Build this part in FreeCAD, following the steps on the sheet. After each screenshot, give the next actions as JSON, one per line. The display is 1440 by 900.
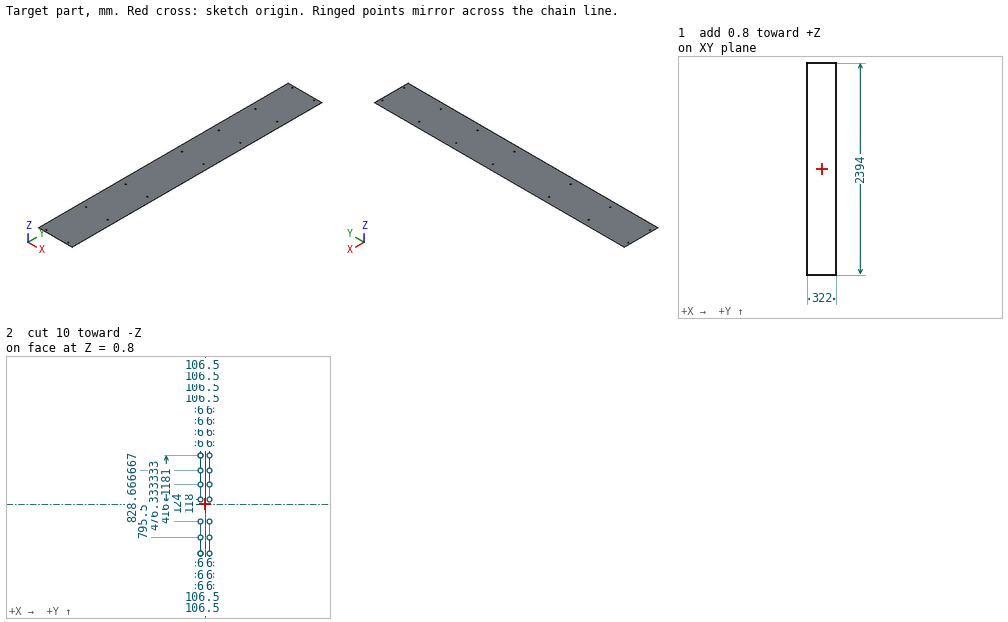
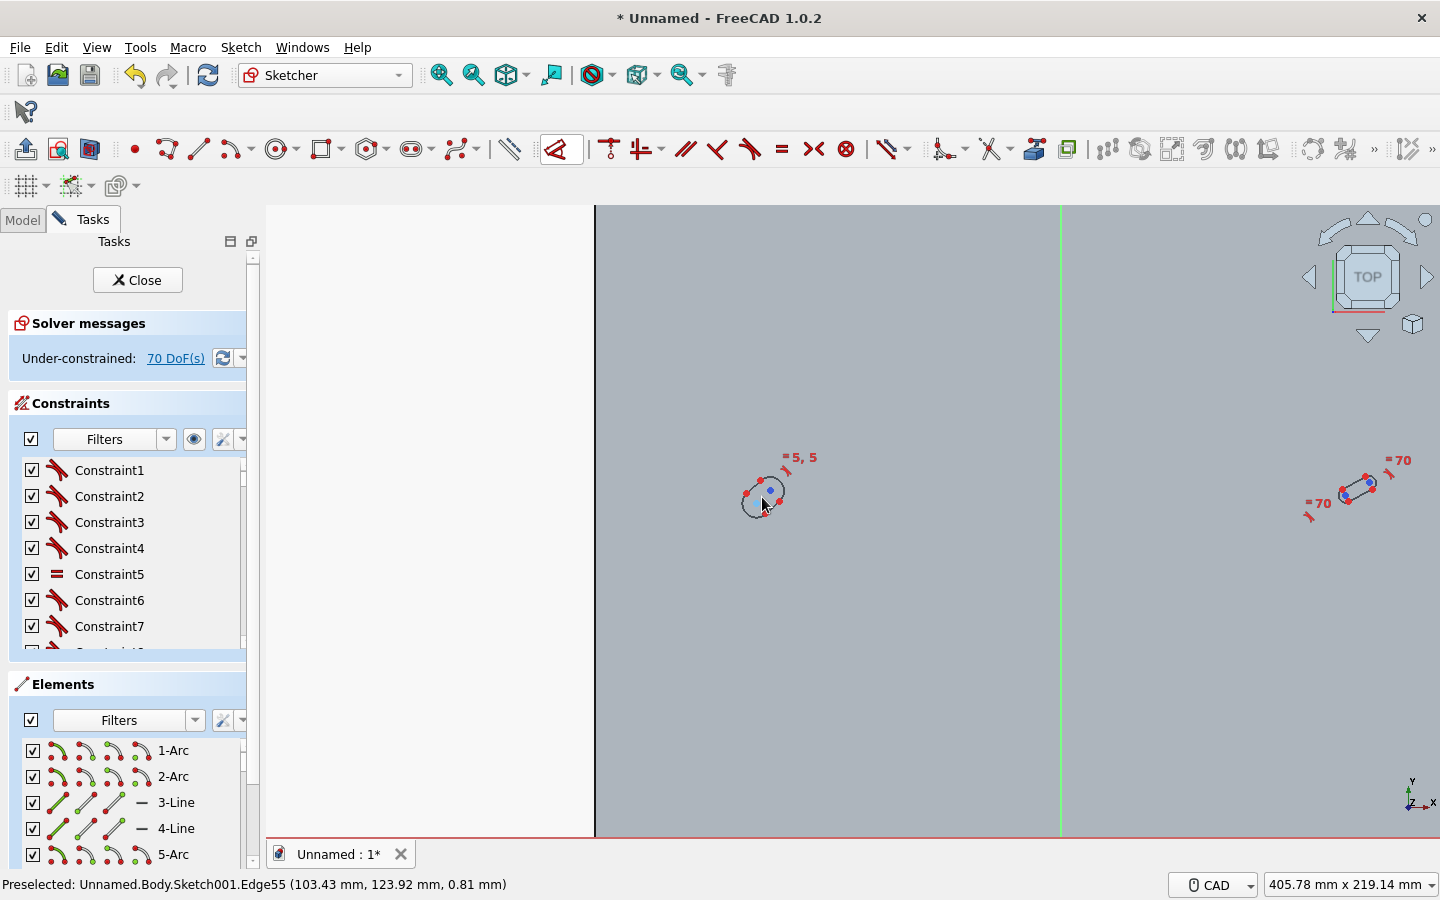
{"action": "left_click", "coordinate": [757, 485]}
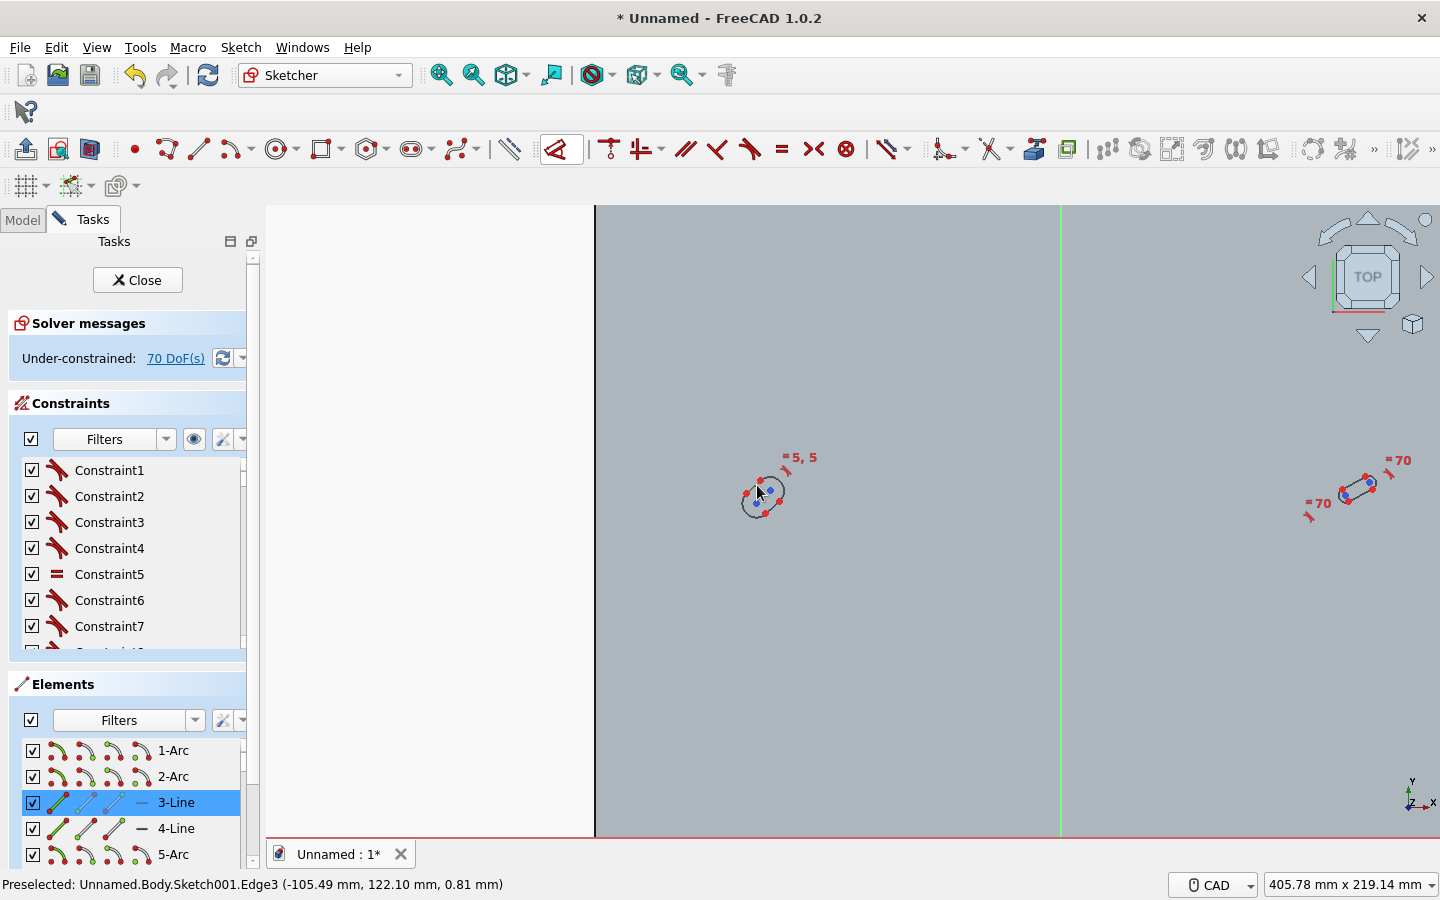
{"action": "key", "text": "h"}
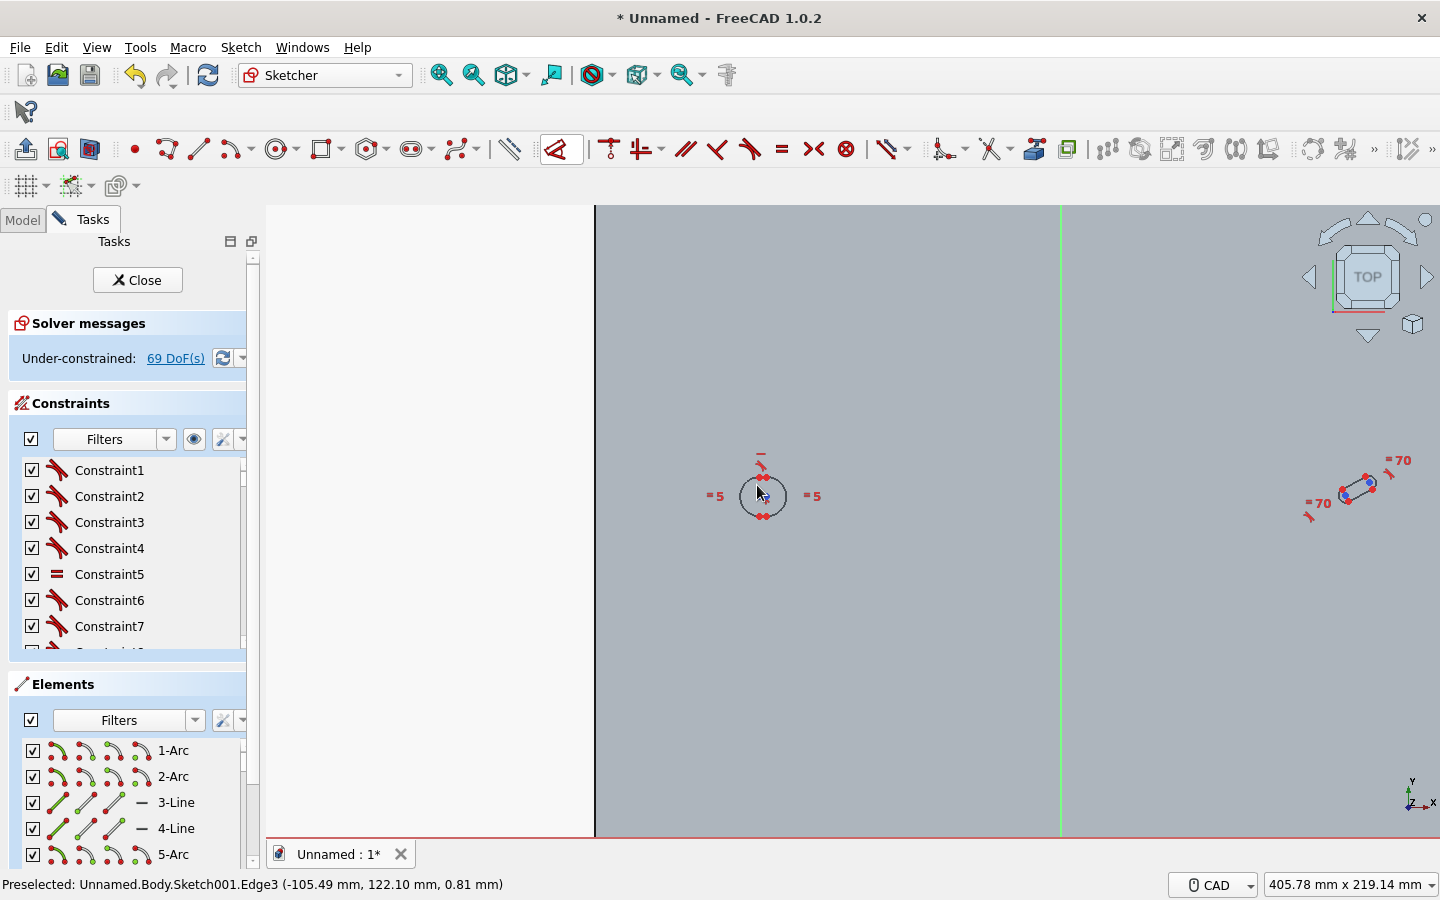
{"action": "scroll", "coordinate": [767, 502], "scroll_direction": "down", "scroll_amount": 14}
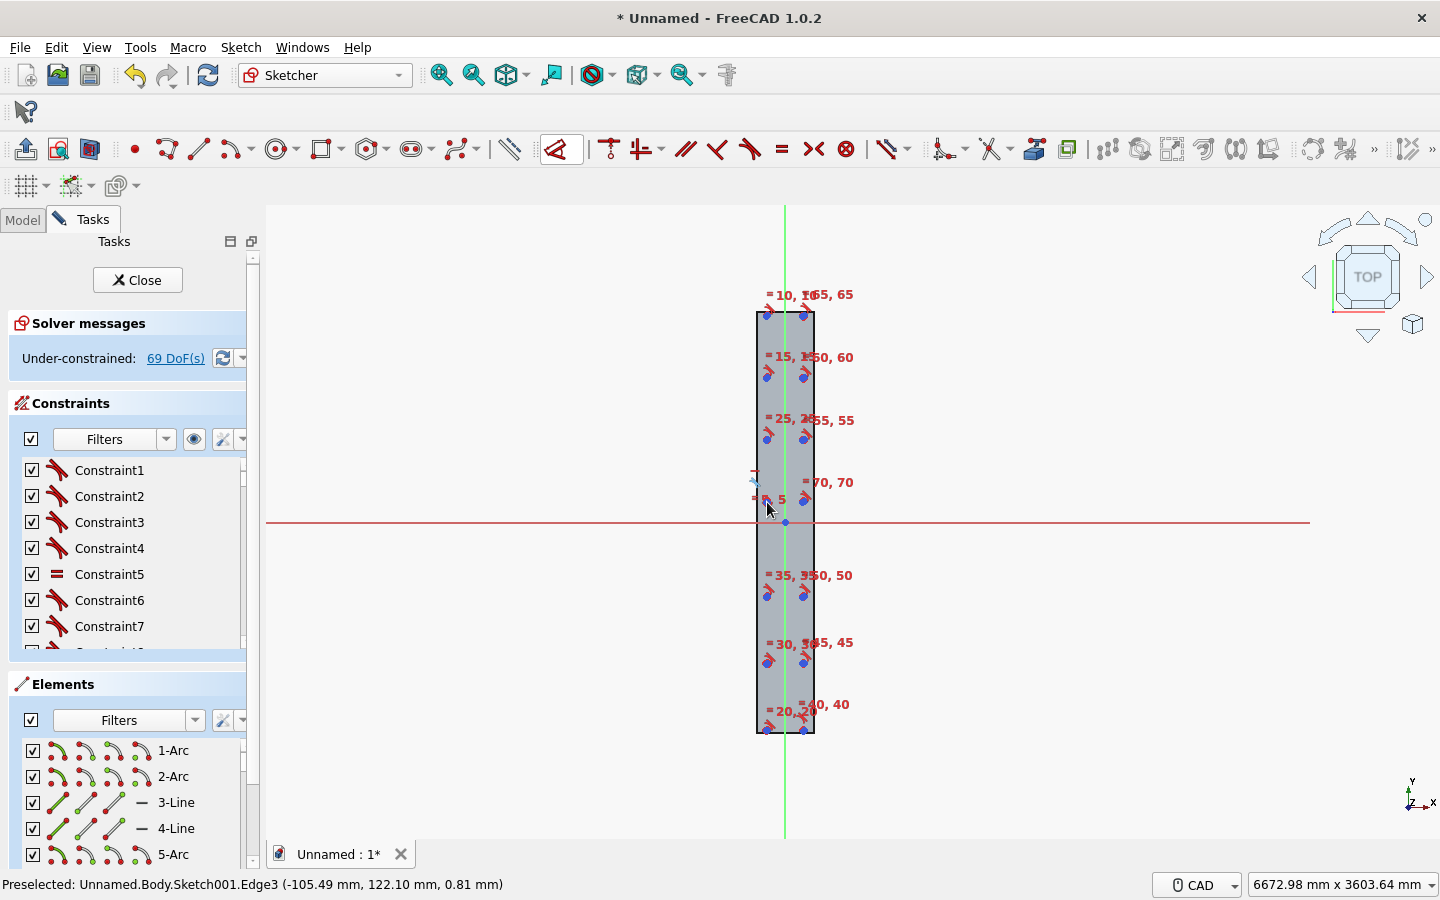
{"action": "scroll", "coordinate": [767, 315], "scroll_direction": "up", "scroll_amount": 14}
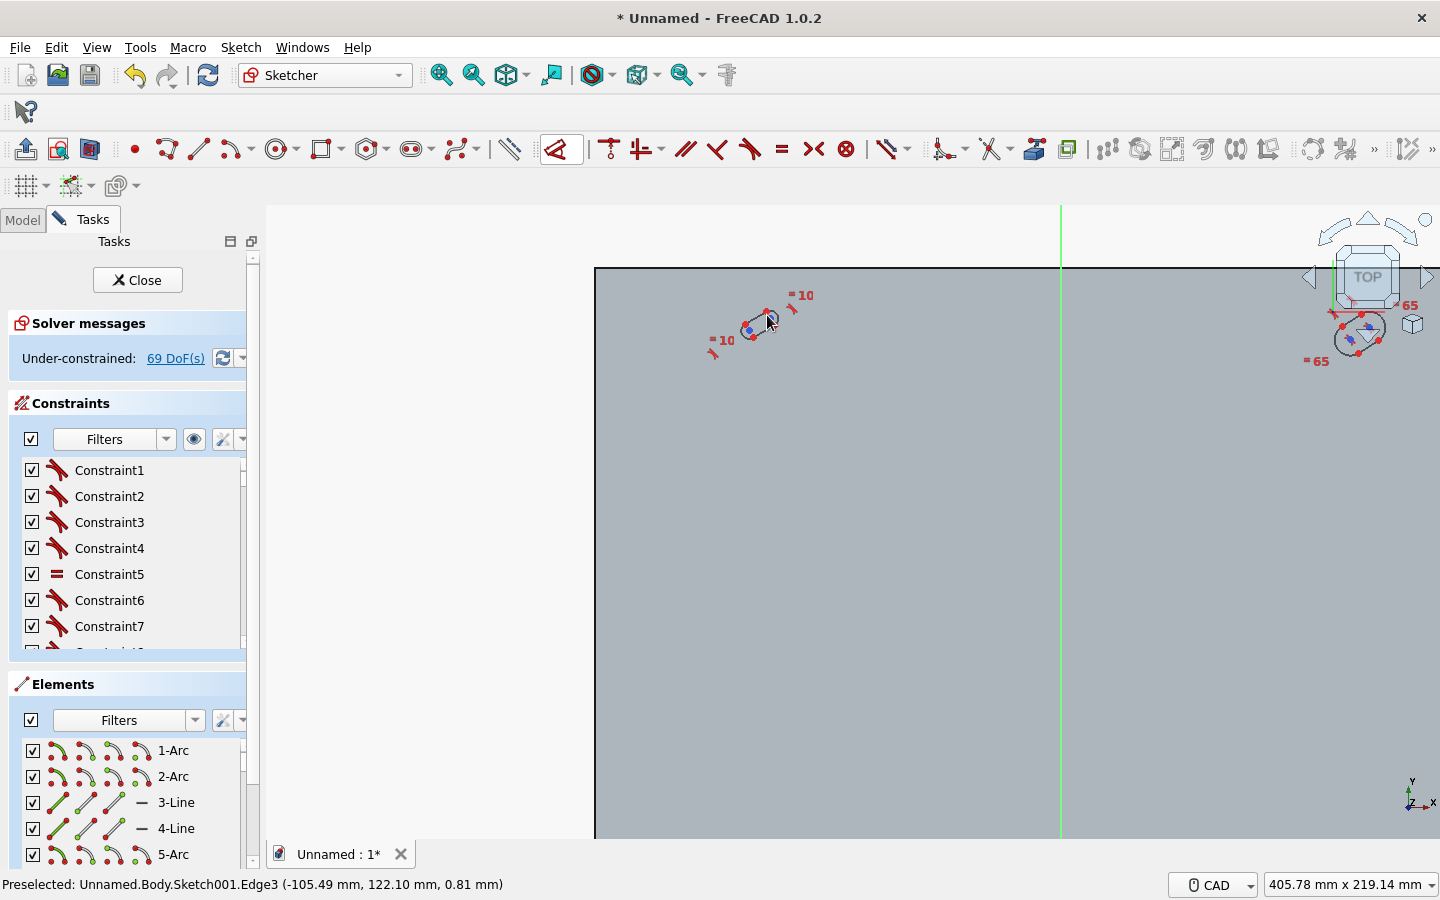
{"action": "left_click", "coordinate": [754, 319]}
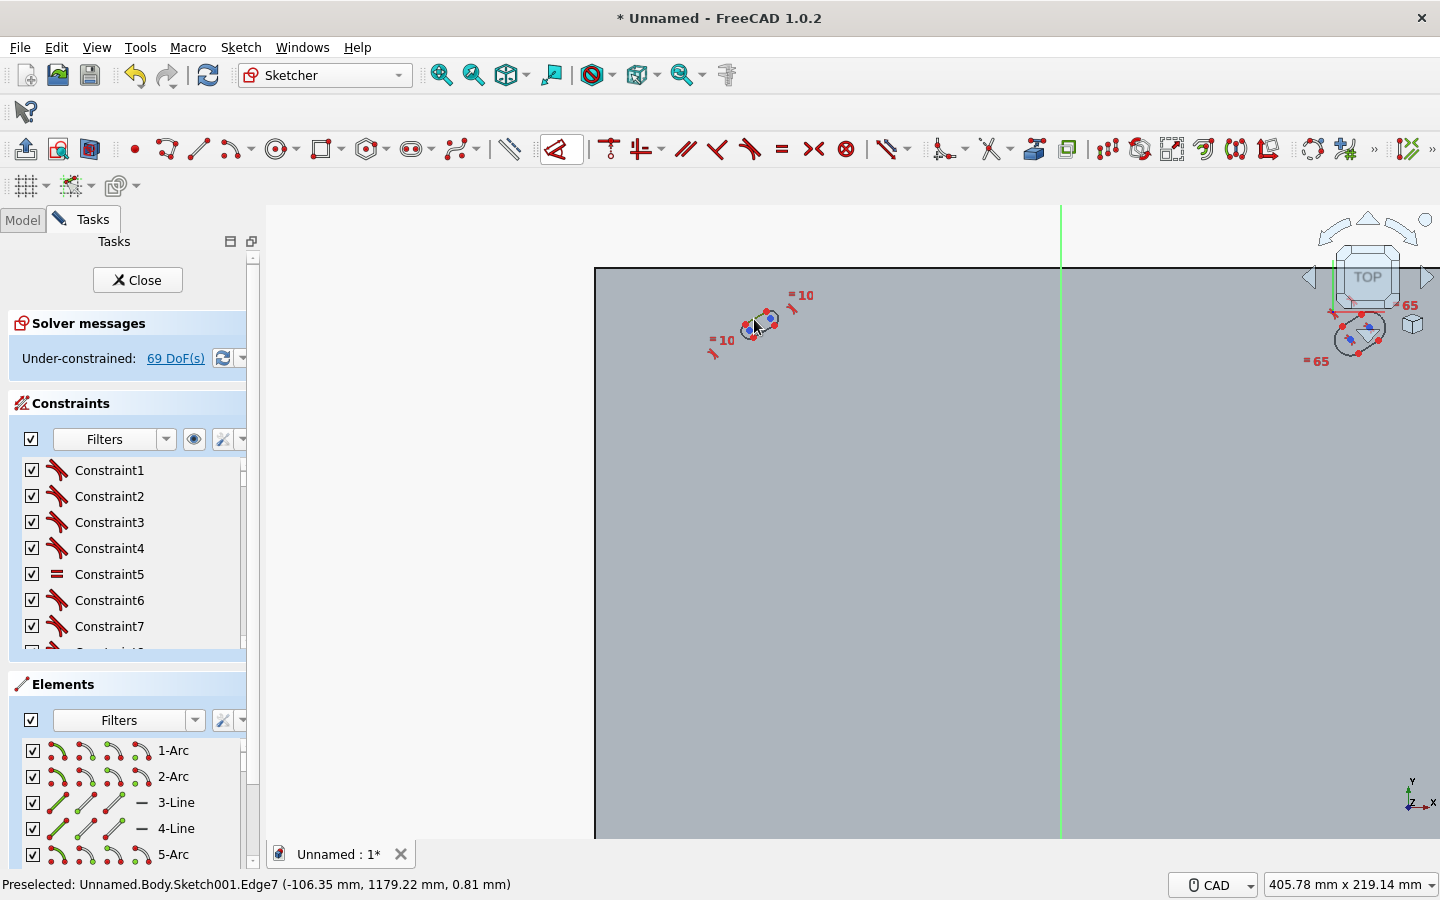
{"action": "key", "text": "h"}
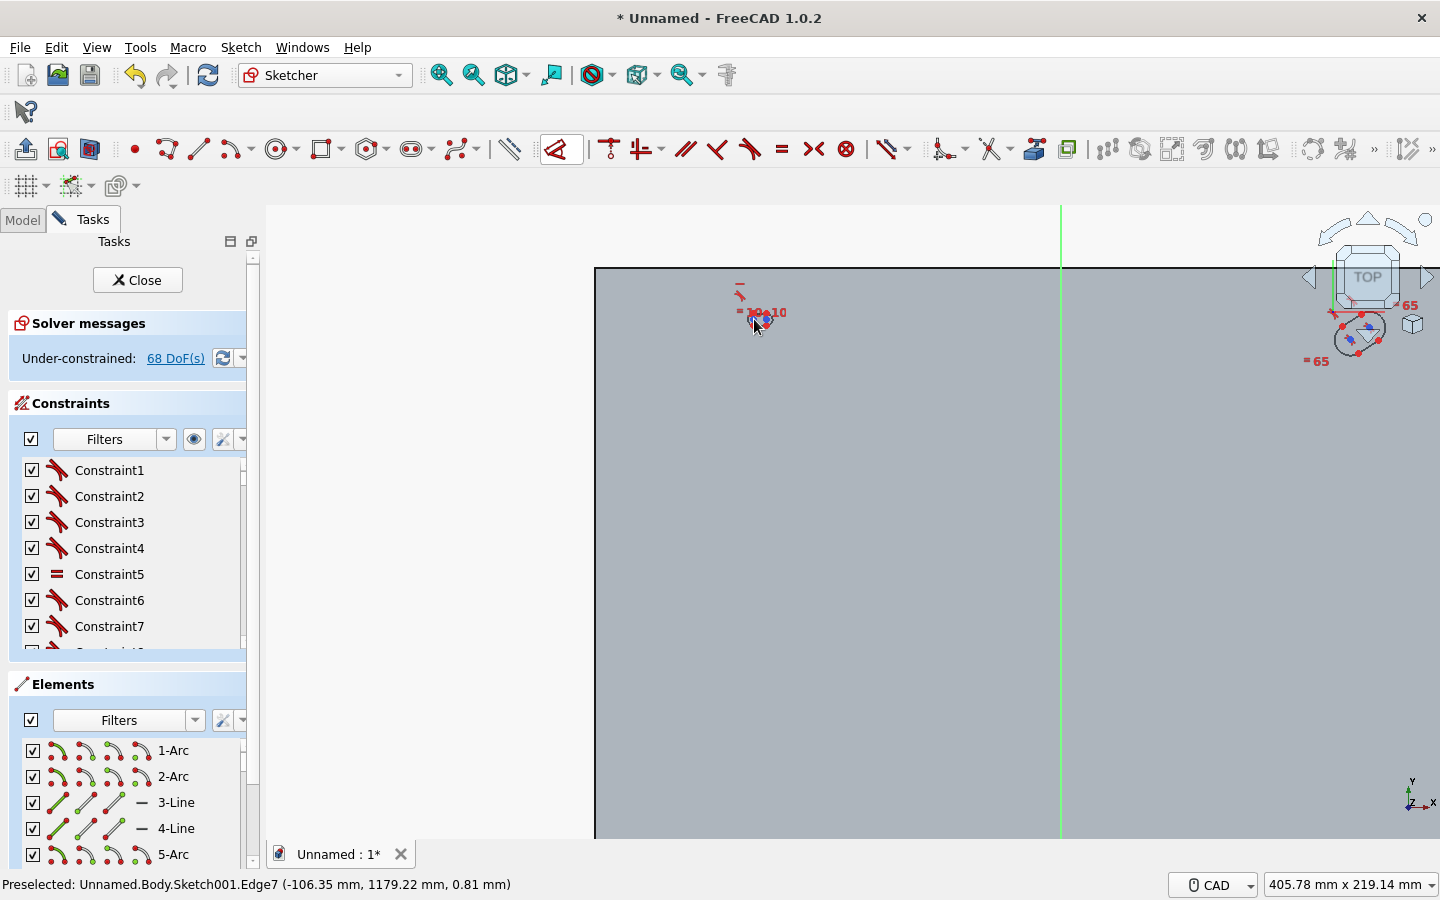
{"action": "scroll", "coordinate": [767, 314], "scroll_direction": "down", "scroll_amount": 14}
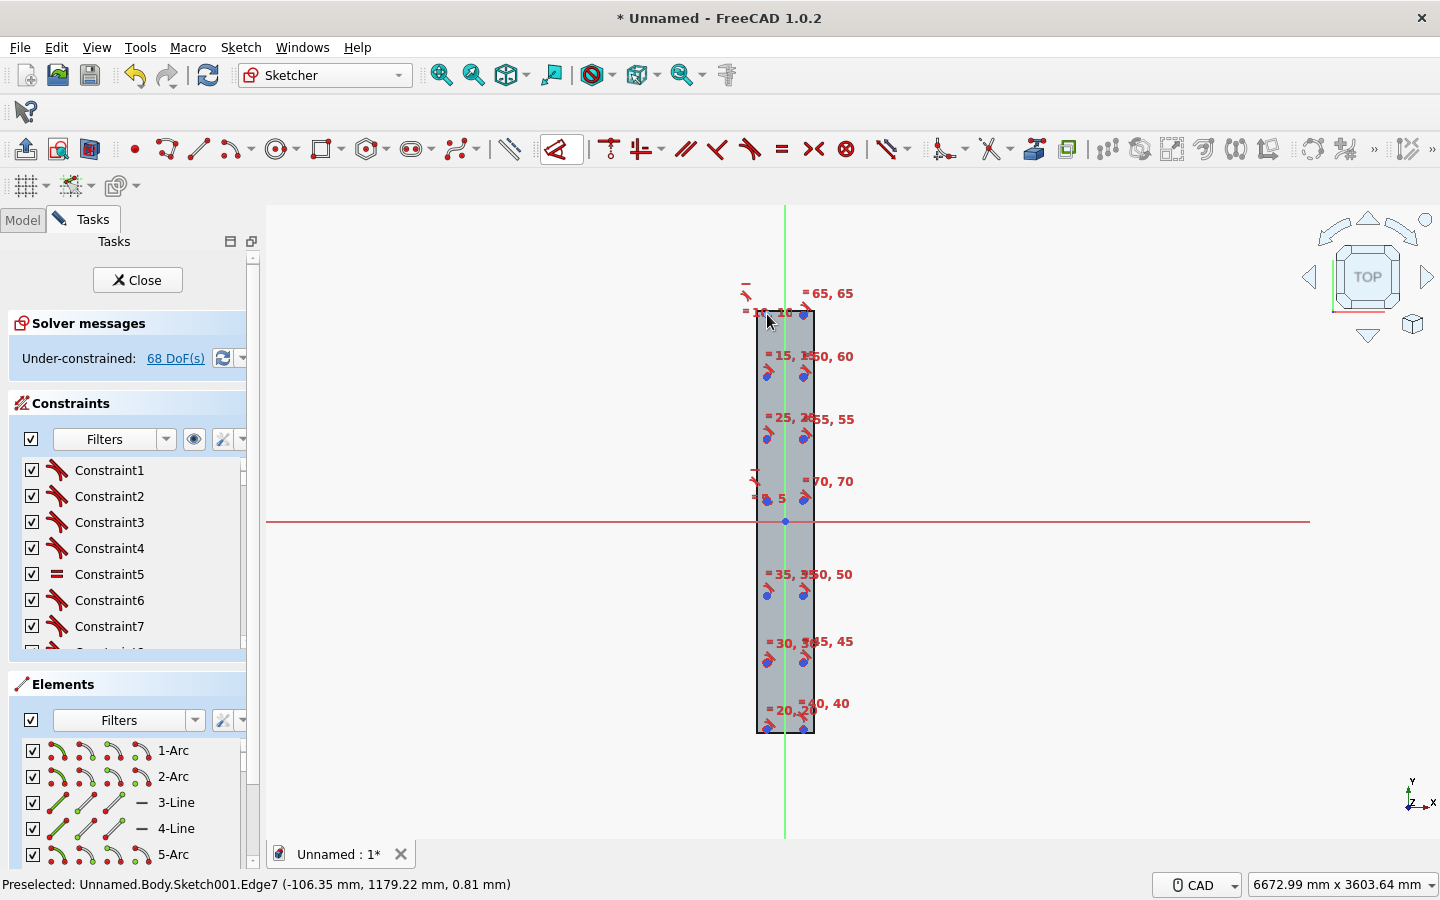
{"action": "scroll", "coordinate": [767, 376], "scroll_direction": "up", "scroll_amount": 14}